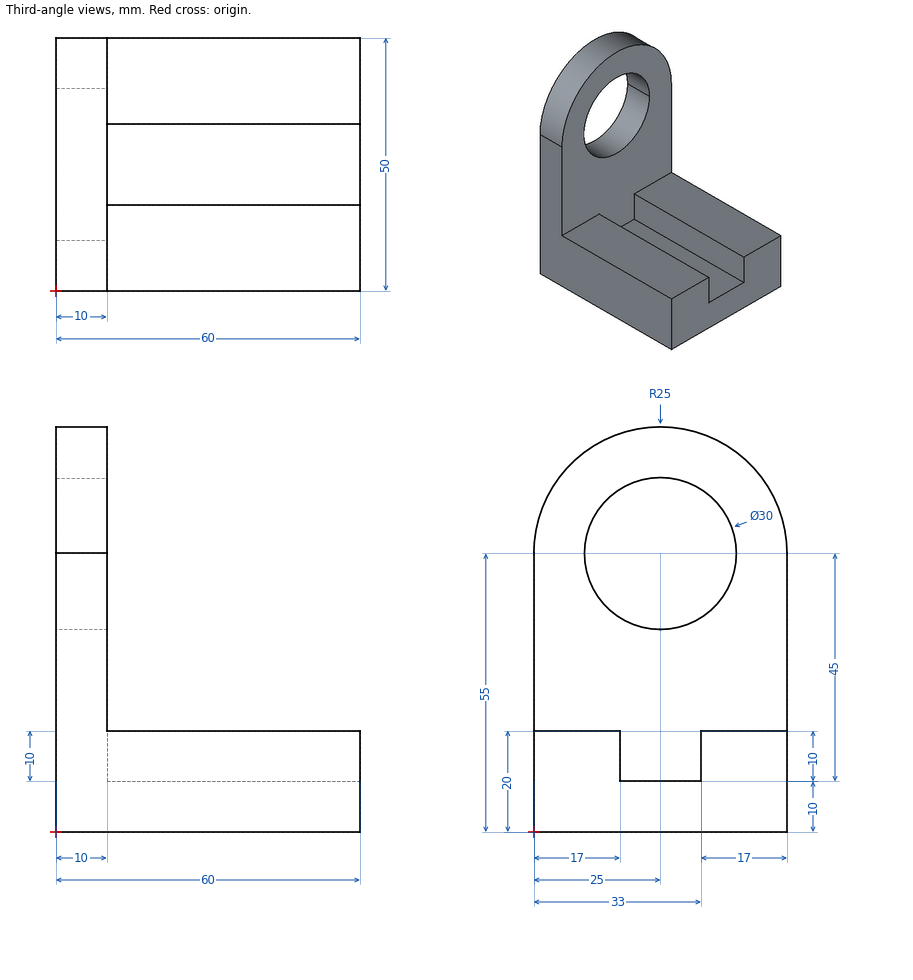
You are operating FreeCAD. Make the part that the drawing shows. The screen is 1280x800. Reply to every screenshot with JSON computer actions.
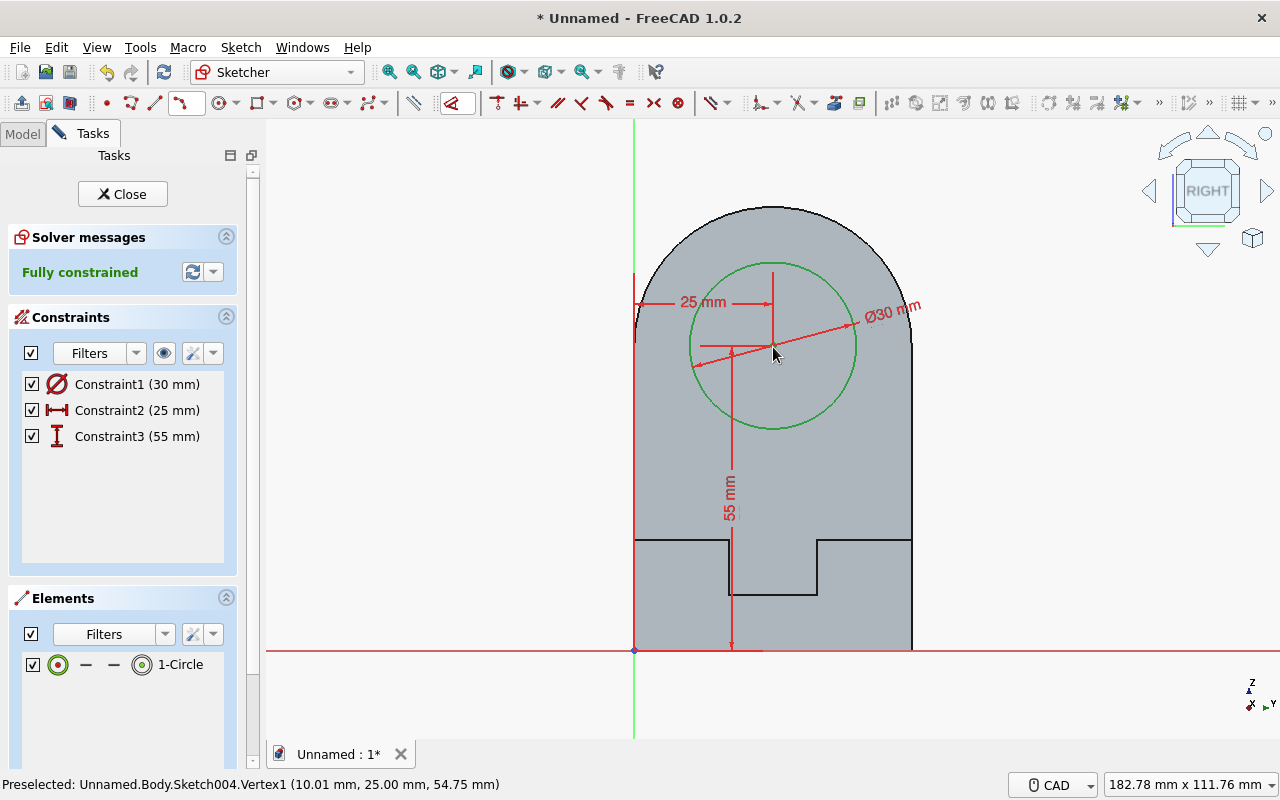
{"action": "left_click", "coordinate": [123, 194]}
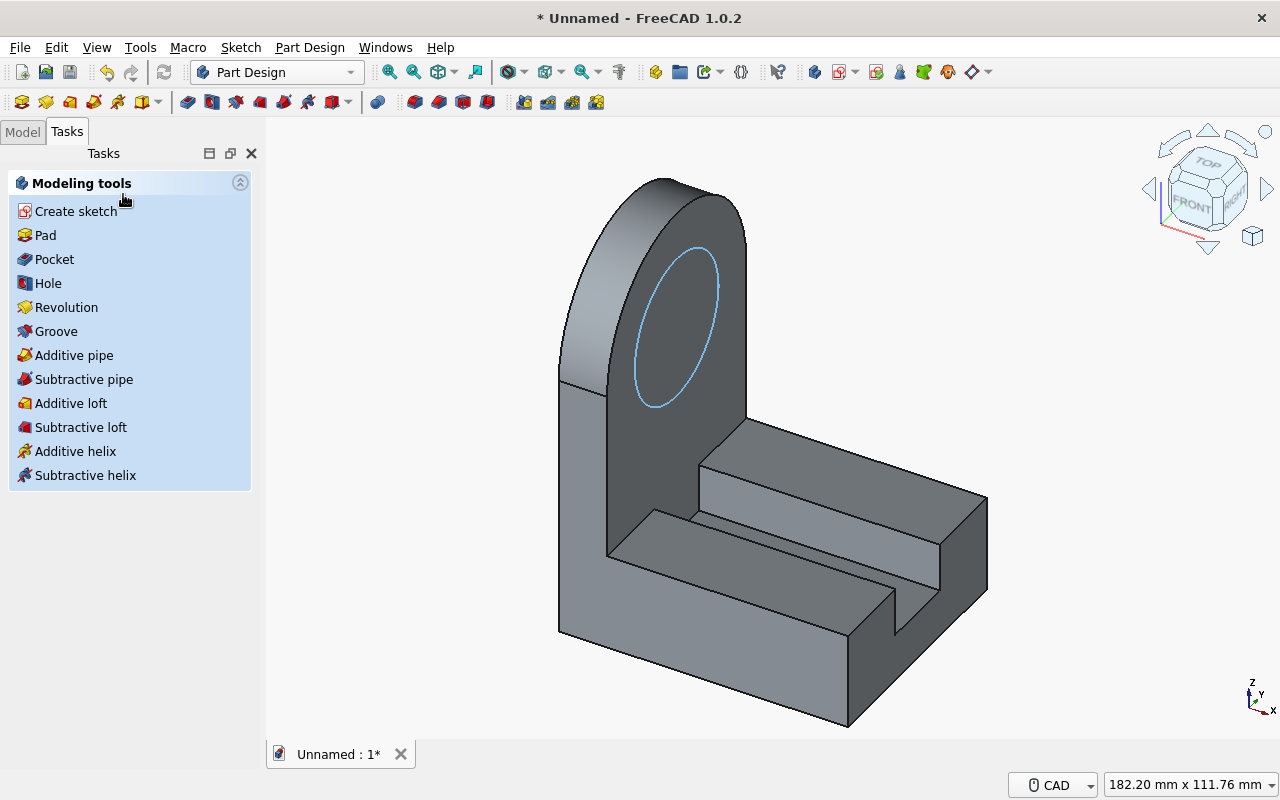
{"action": "left_click", "coordinate": [188, 102]}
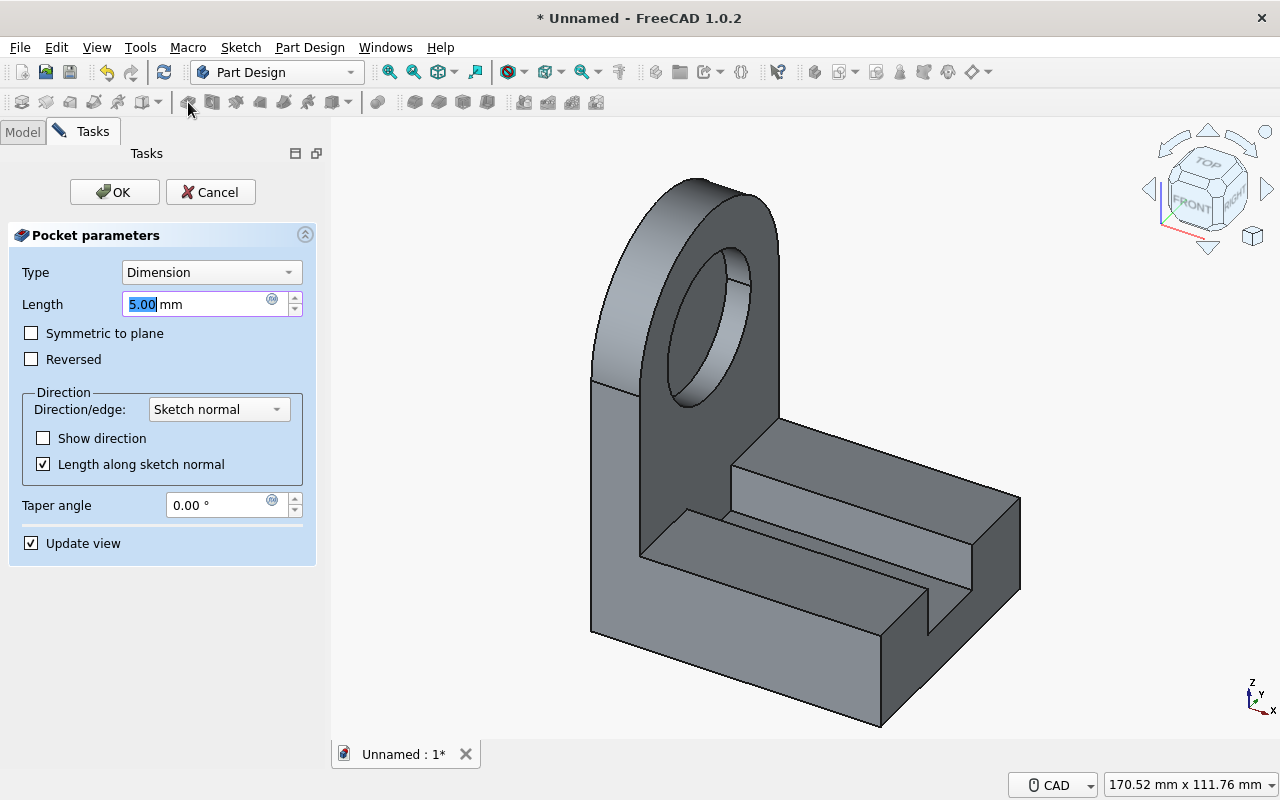
{"action": "type", "text": "10"}
{"action": "key", "text": "Tab"}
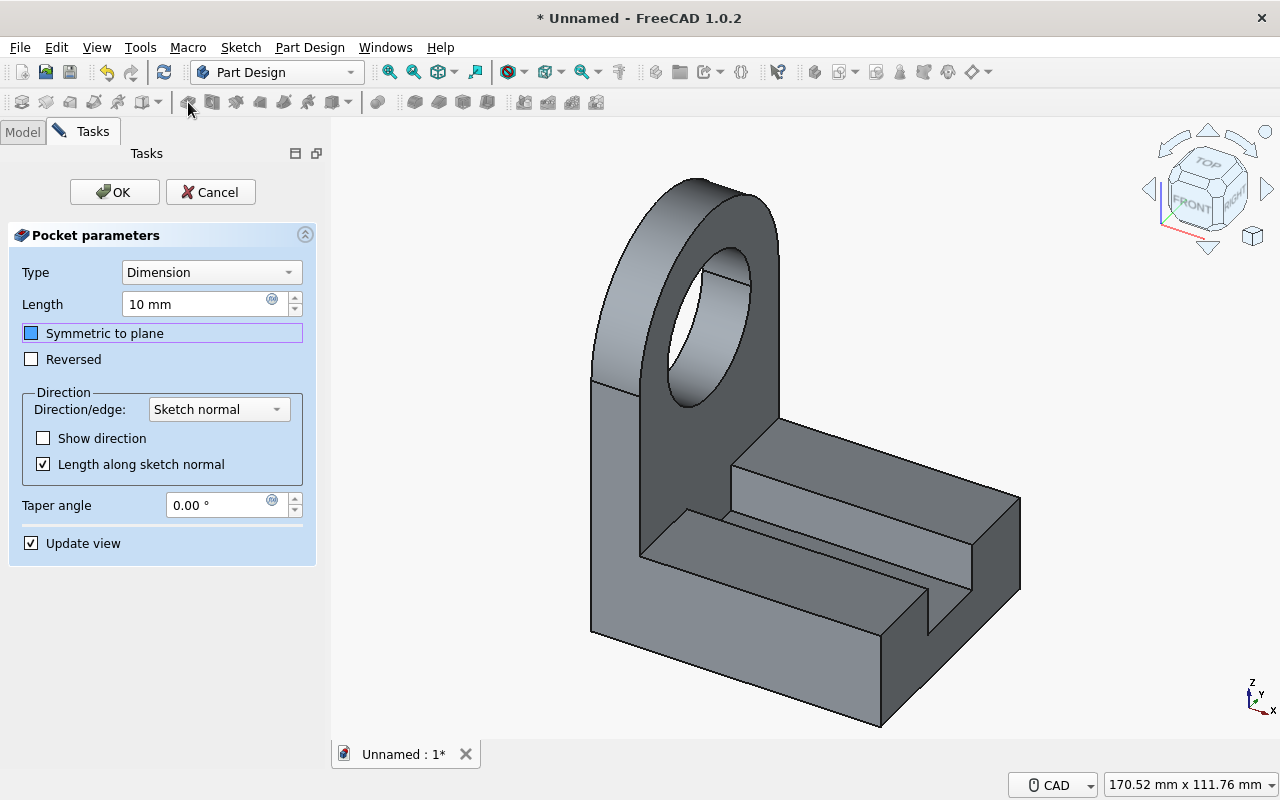
{"action": "left_click", "coordinate": [115, 192]}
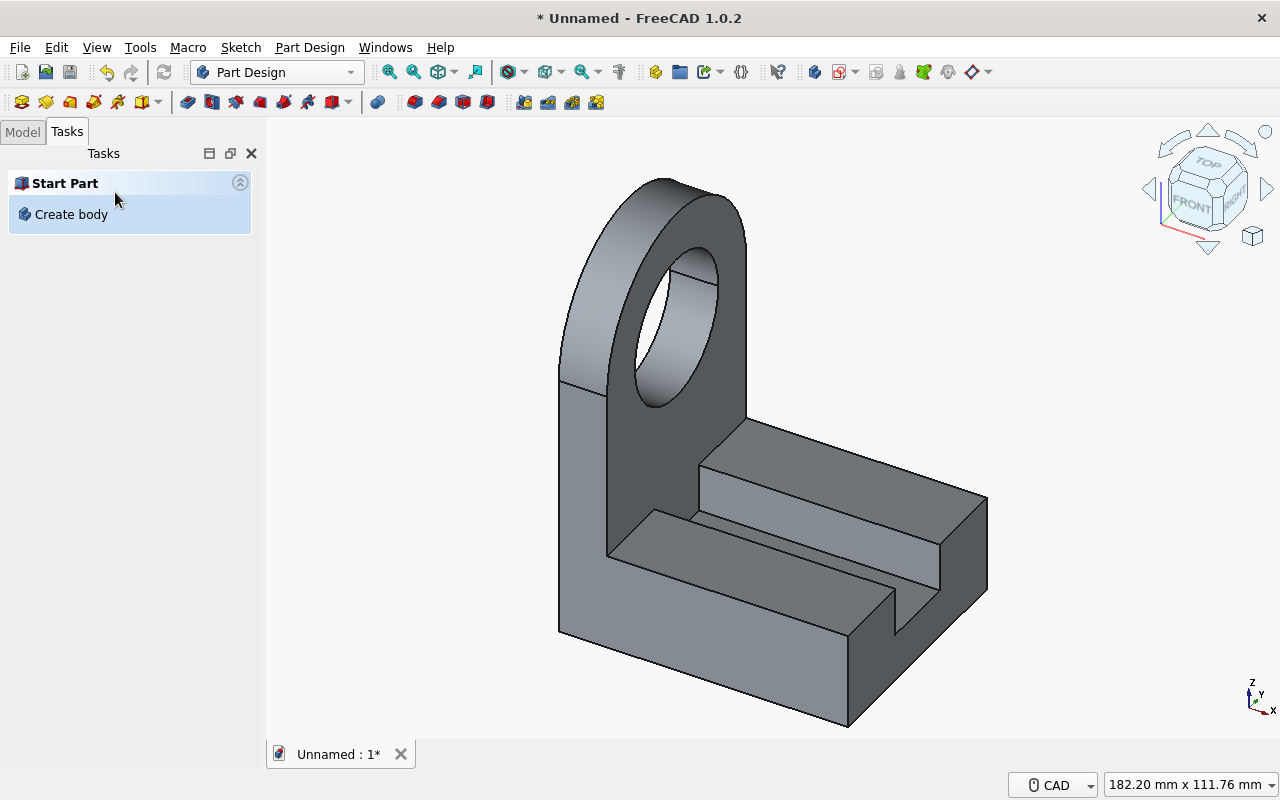
{"action": "key", "text": "0"}